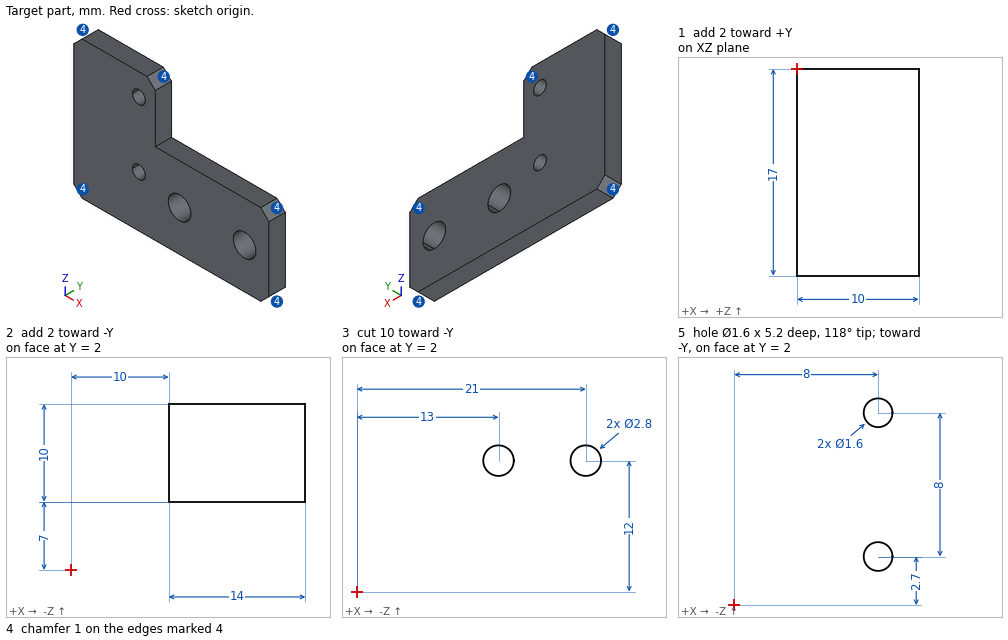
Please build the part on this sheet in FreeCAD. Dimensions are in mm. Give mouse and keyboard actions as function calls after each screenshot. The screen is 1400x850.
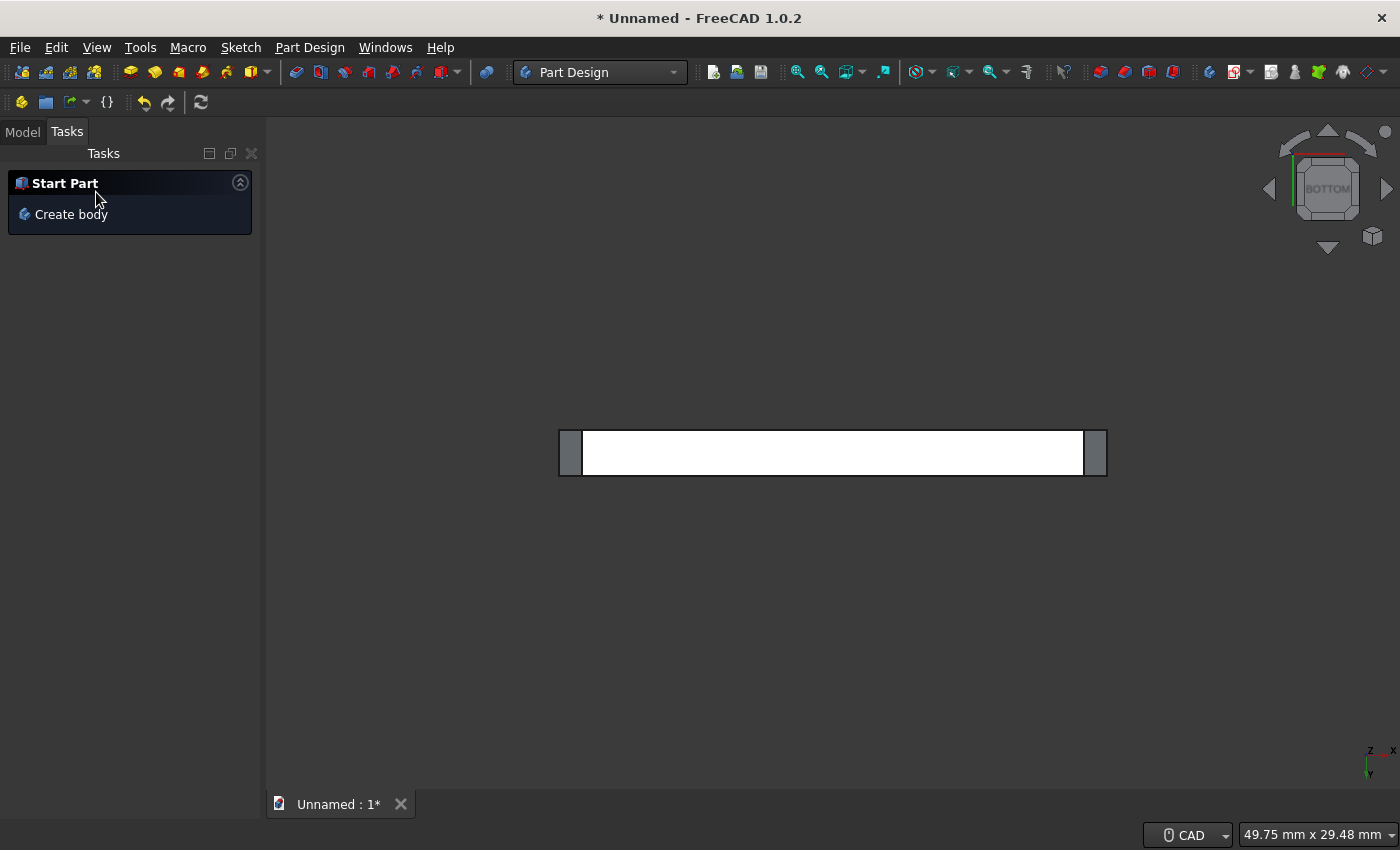
key(4)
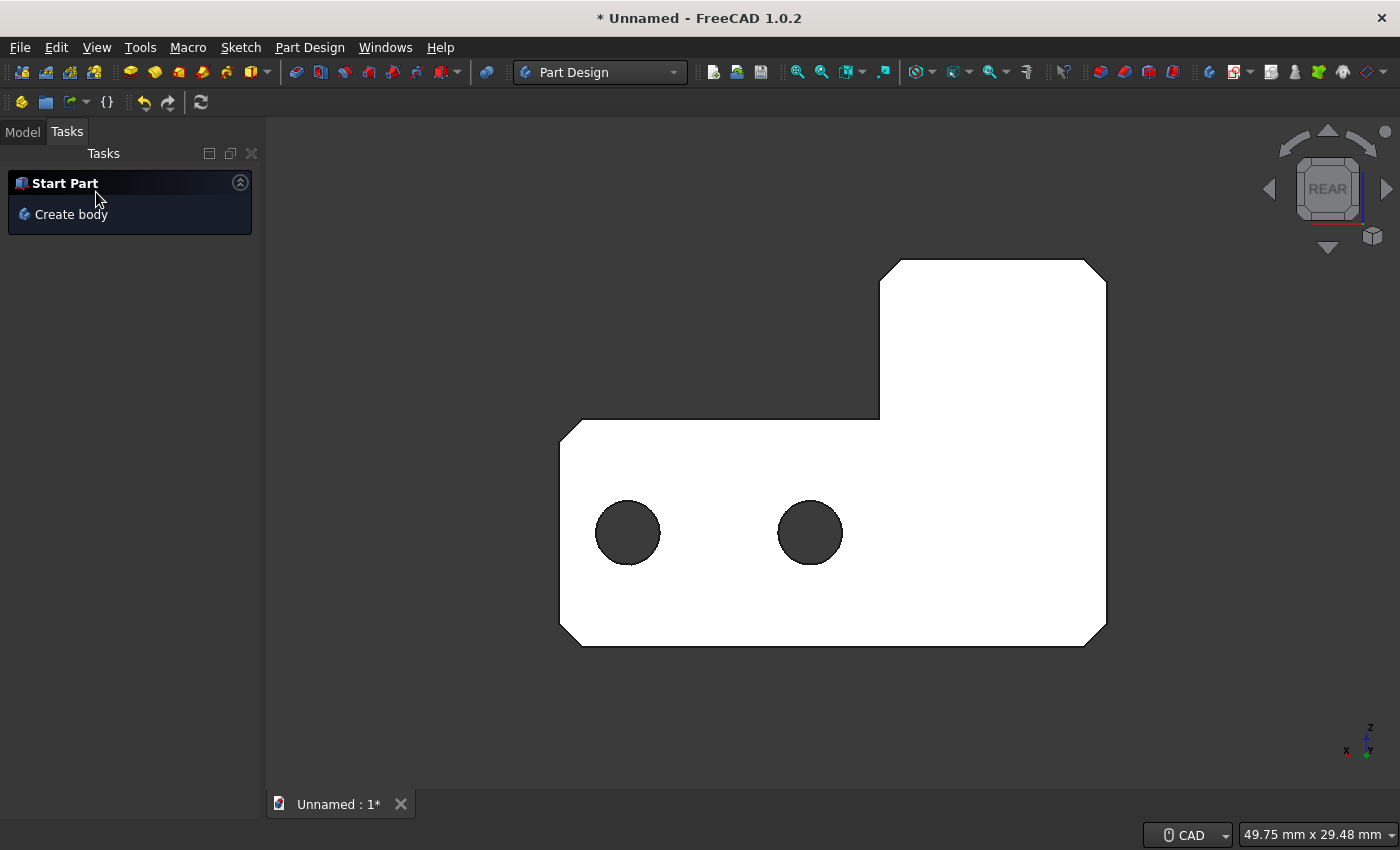
click(989, 507)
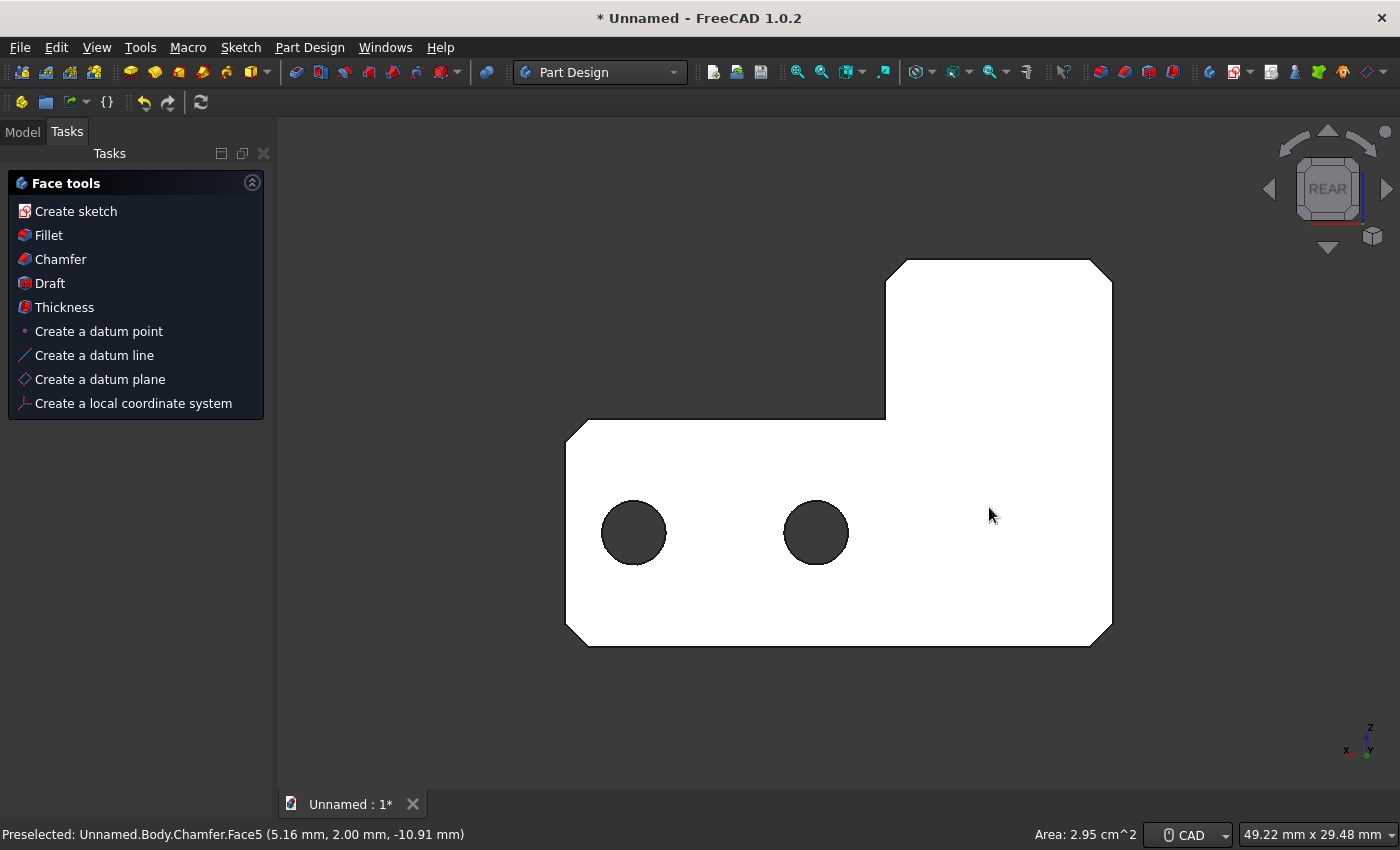
click(1234, 72)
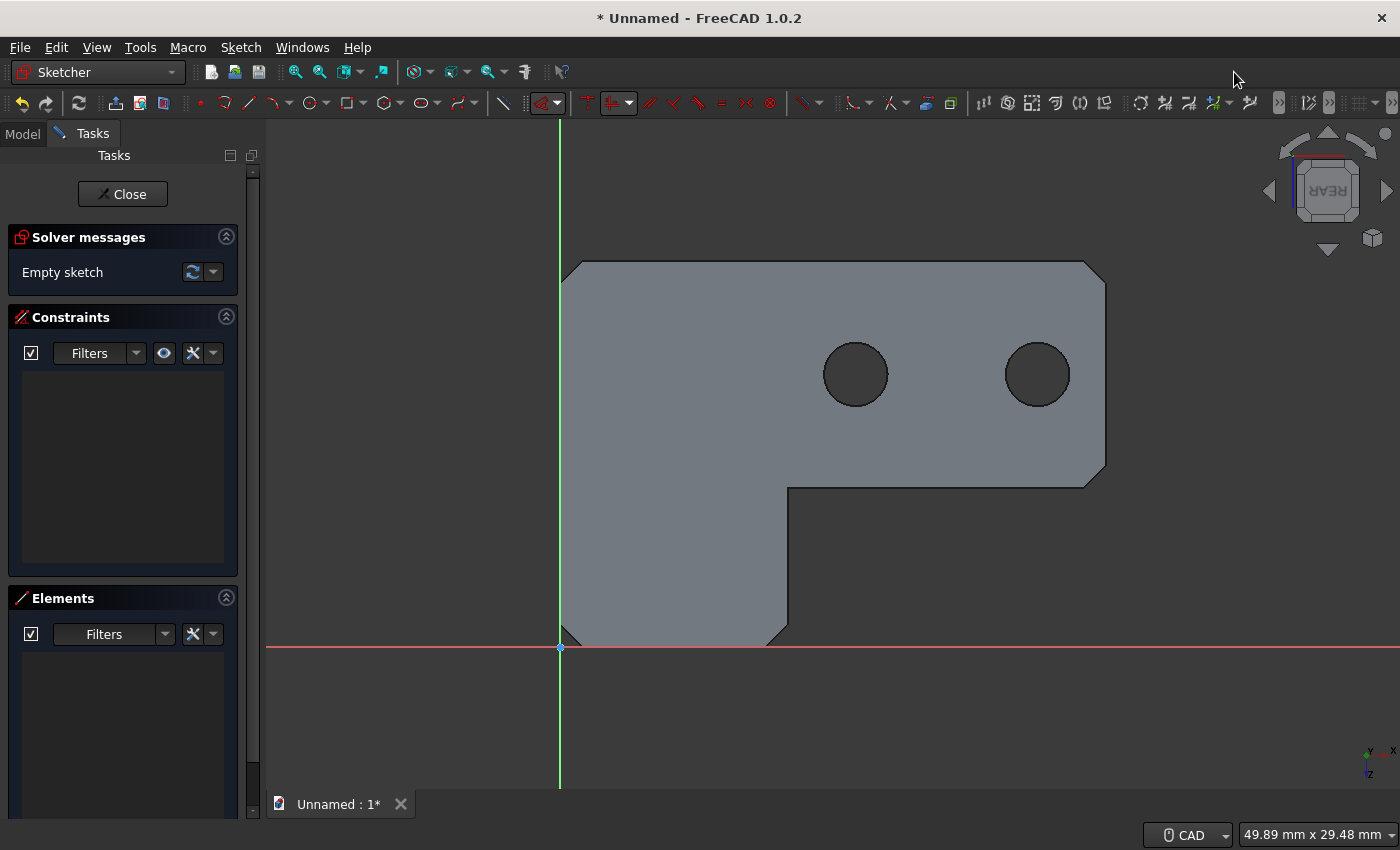
scroll(533, 593, up, 3)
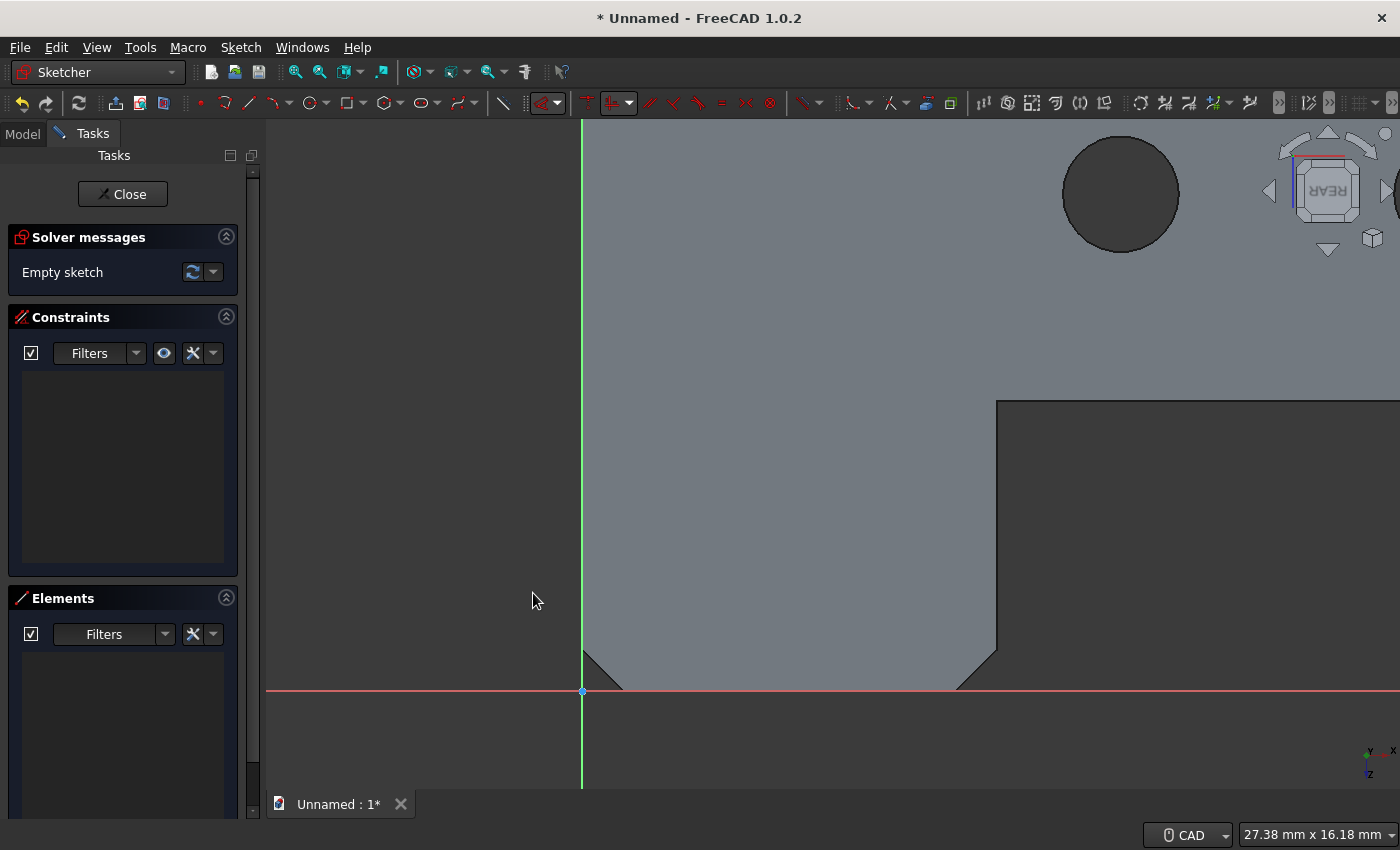
click(310, 104)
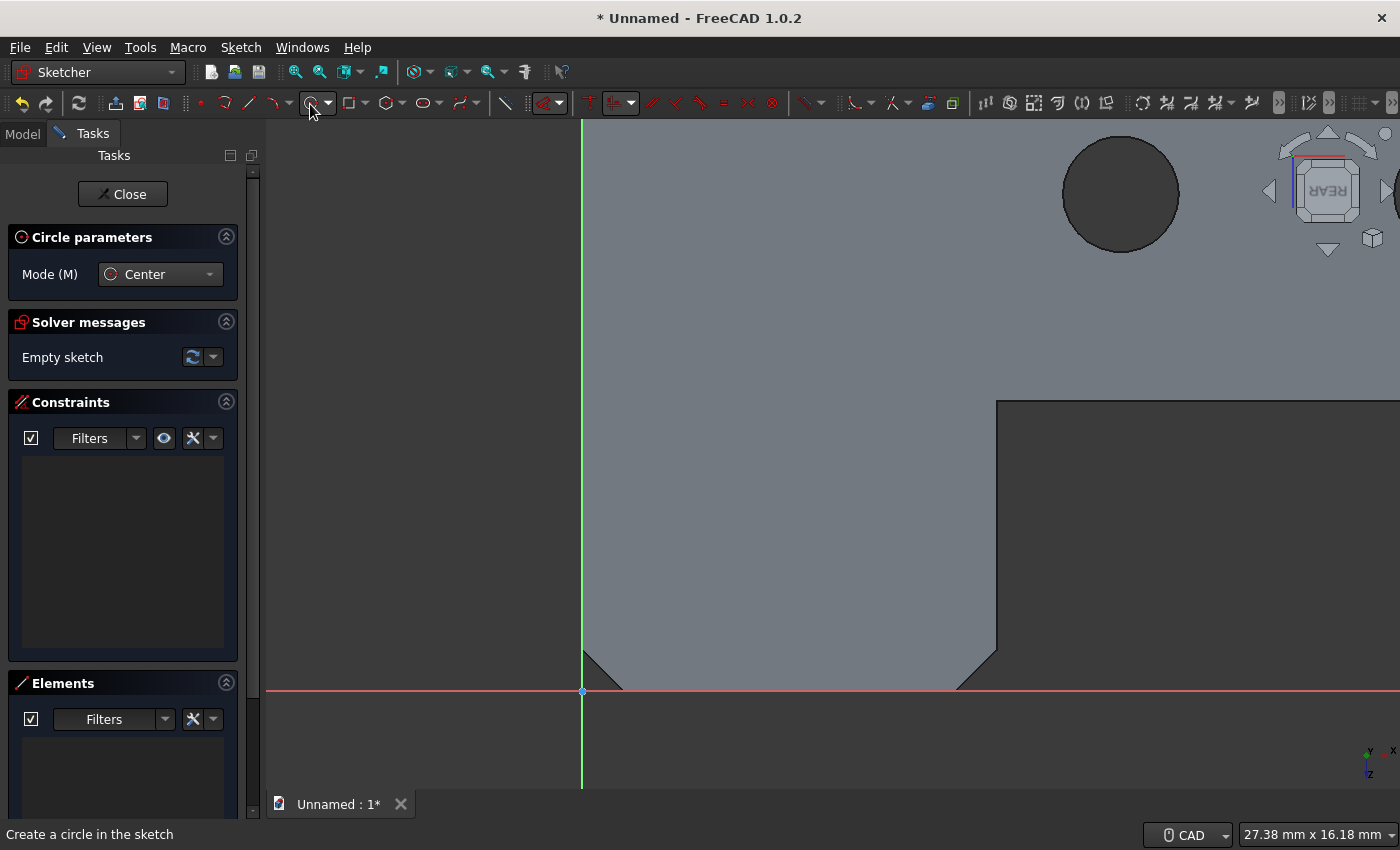
click(914, 248)
click(937, 225)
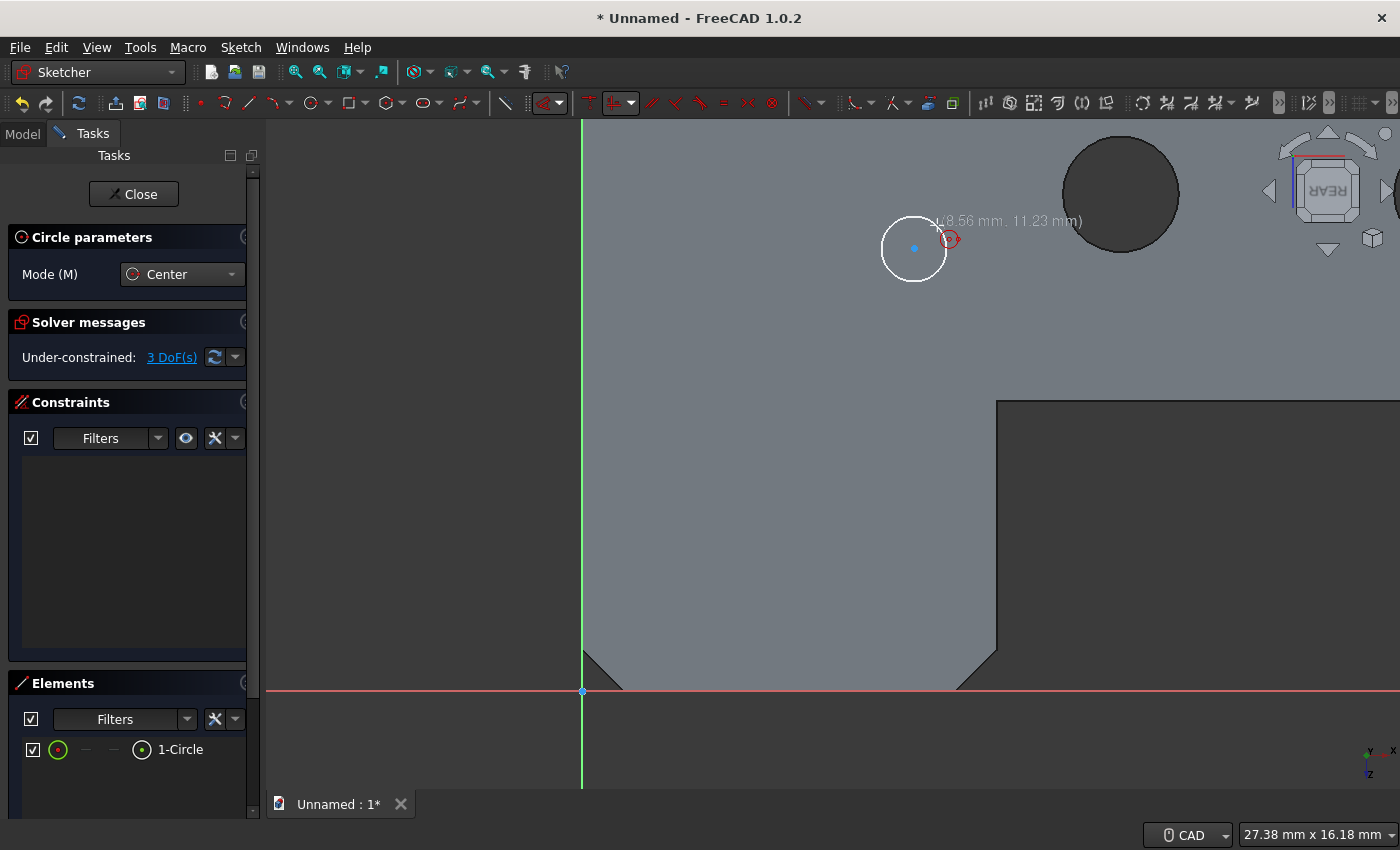
click(914, 579)
click(937, 556)
key(Escape)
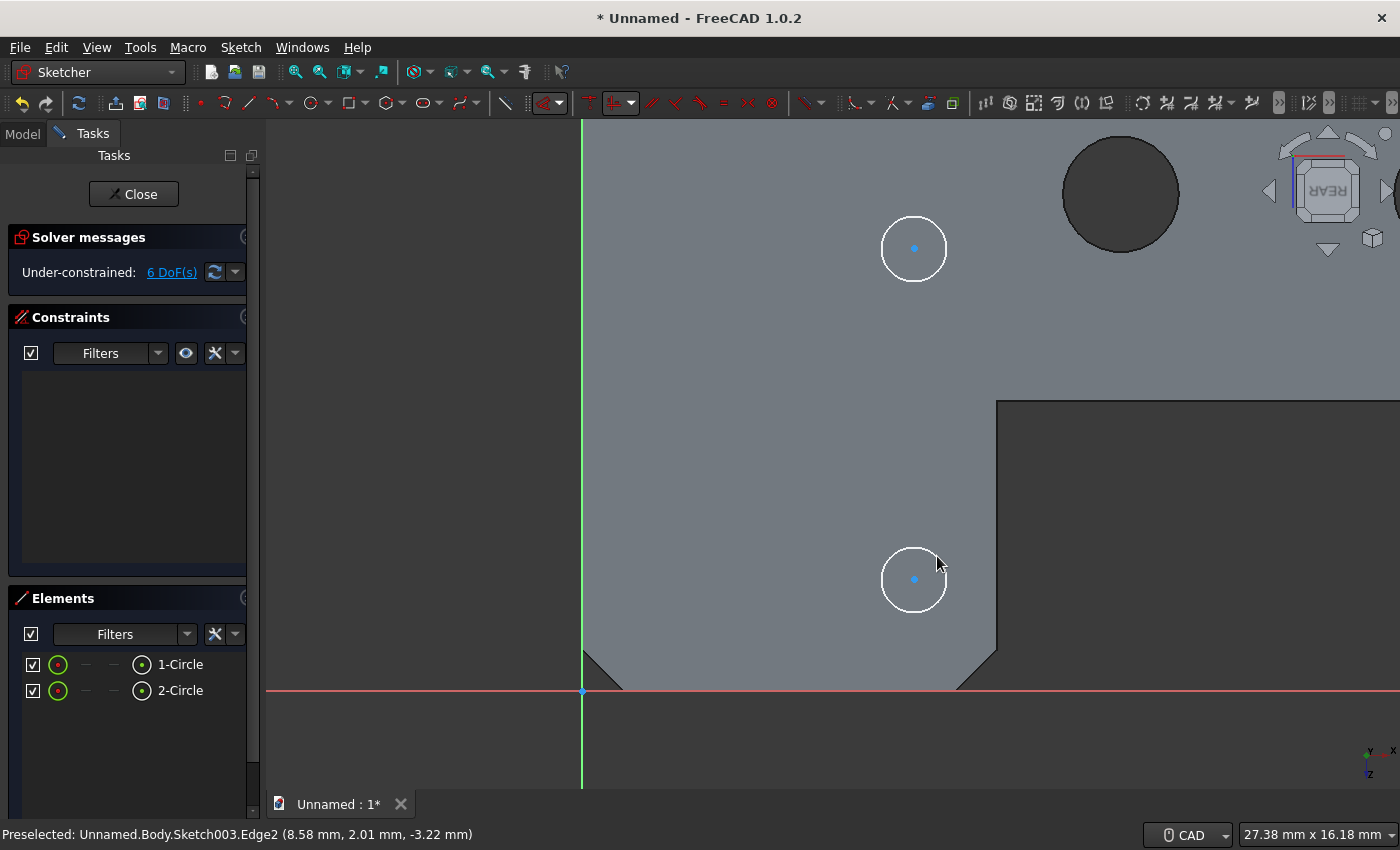
click(937, 226)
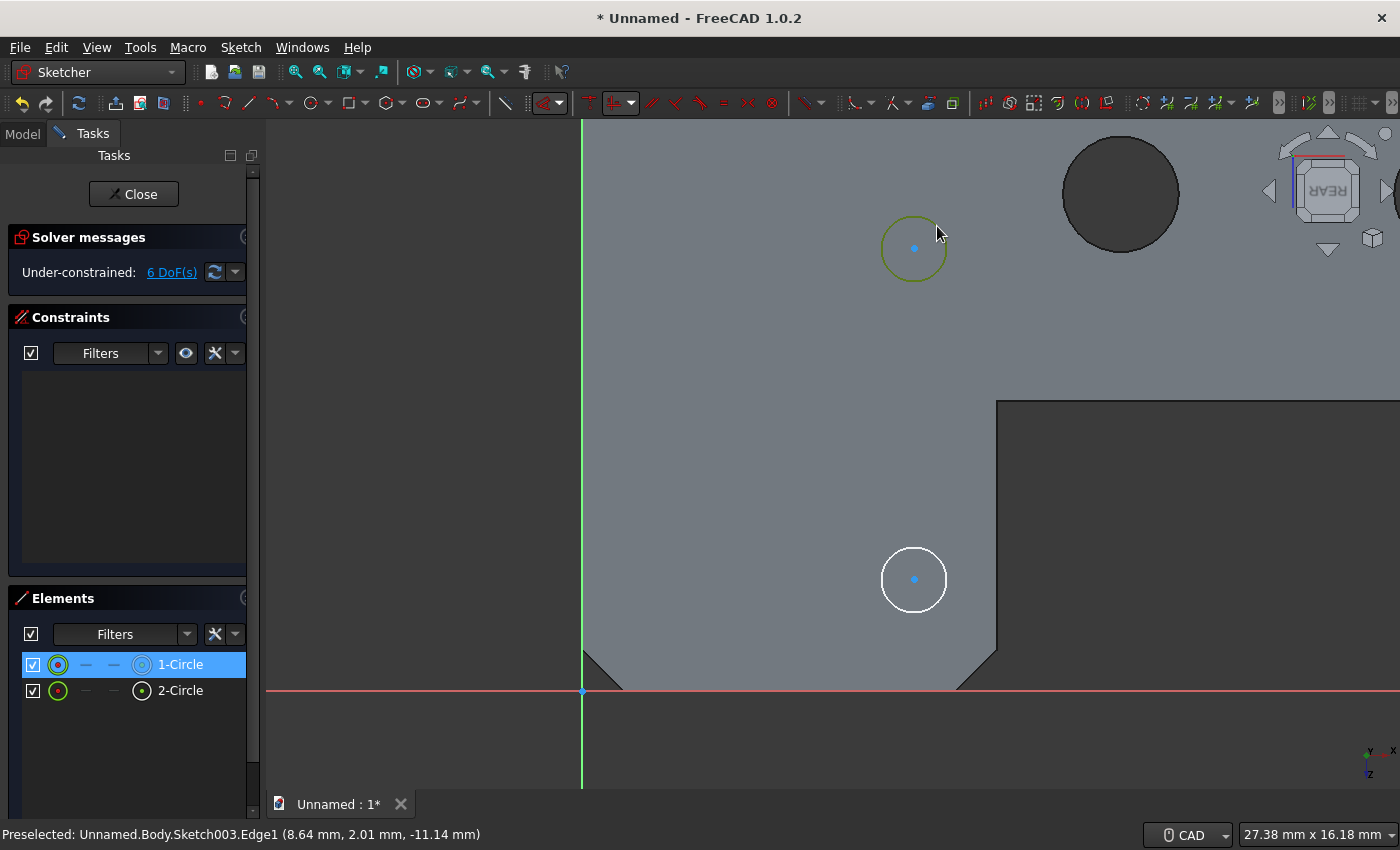
click(937, 557)